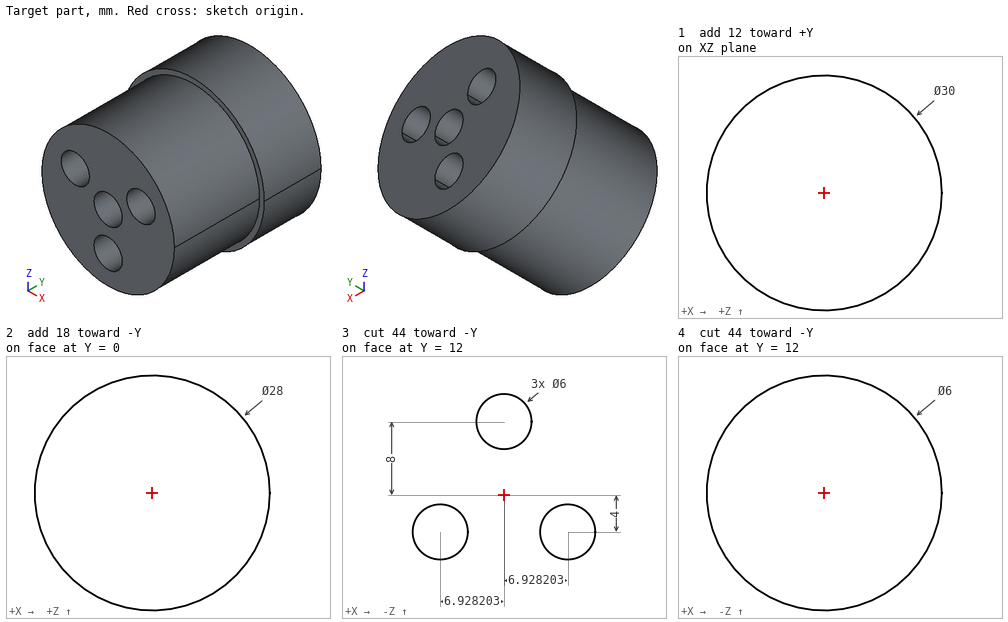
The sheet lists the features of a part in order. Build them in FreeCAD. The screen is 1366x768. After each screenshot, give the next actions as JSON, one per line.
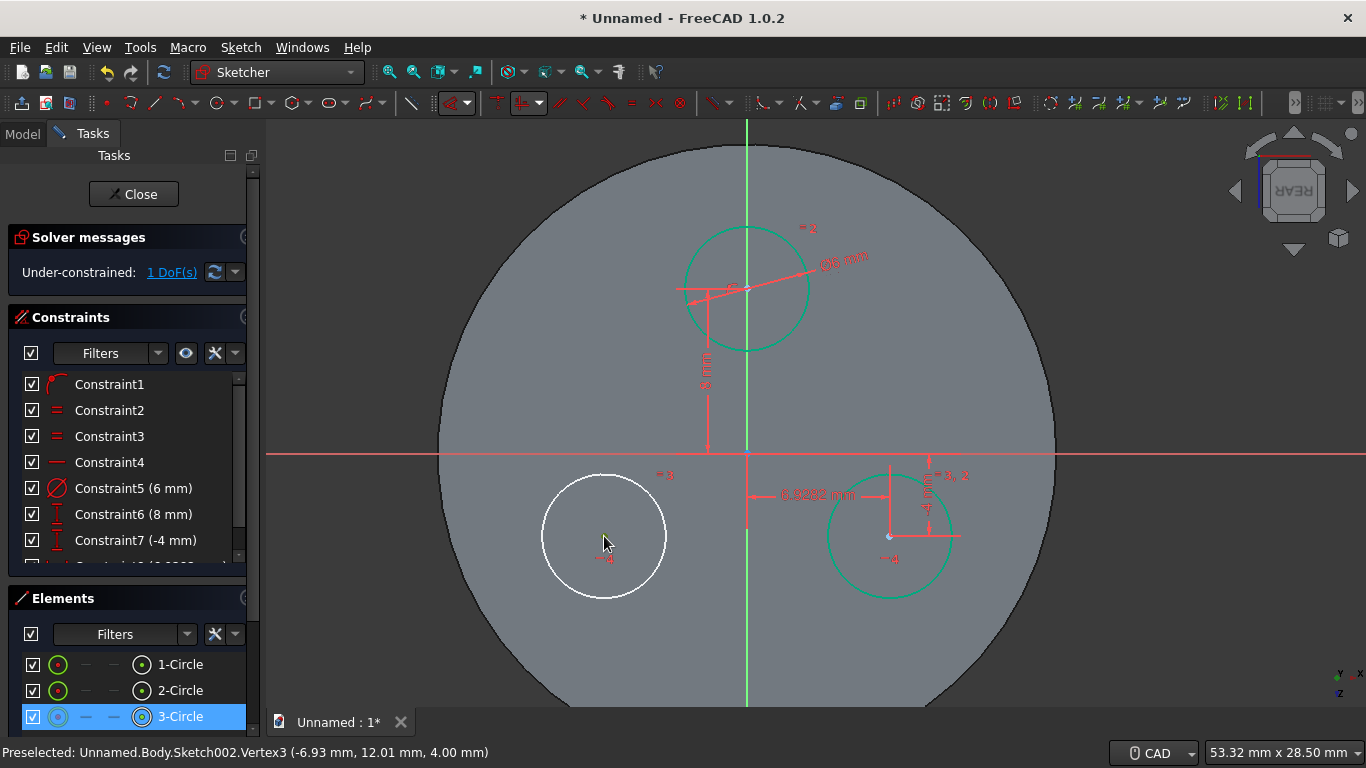
{"action": "left_click", "coordinate": [470, 104]}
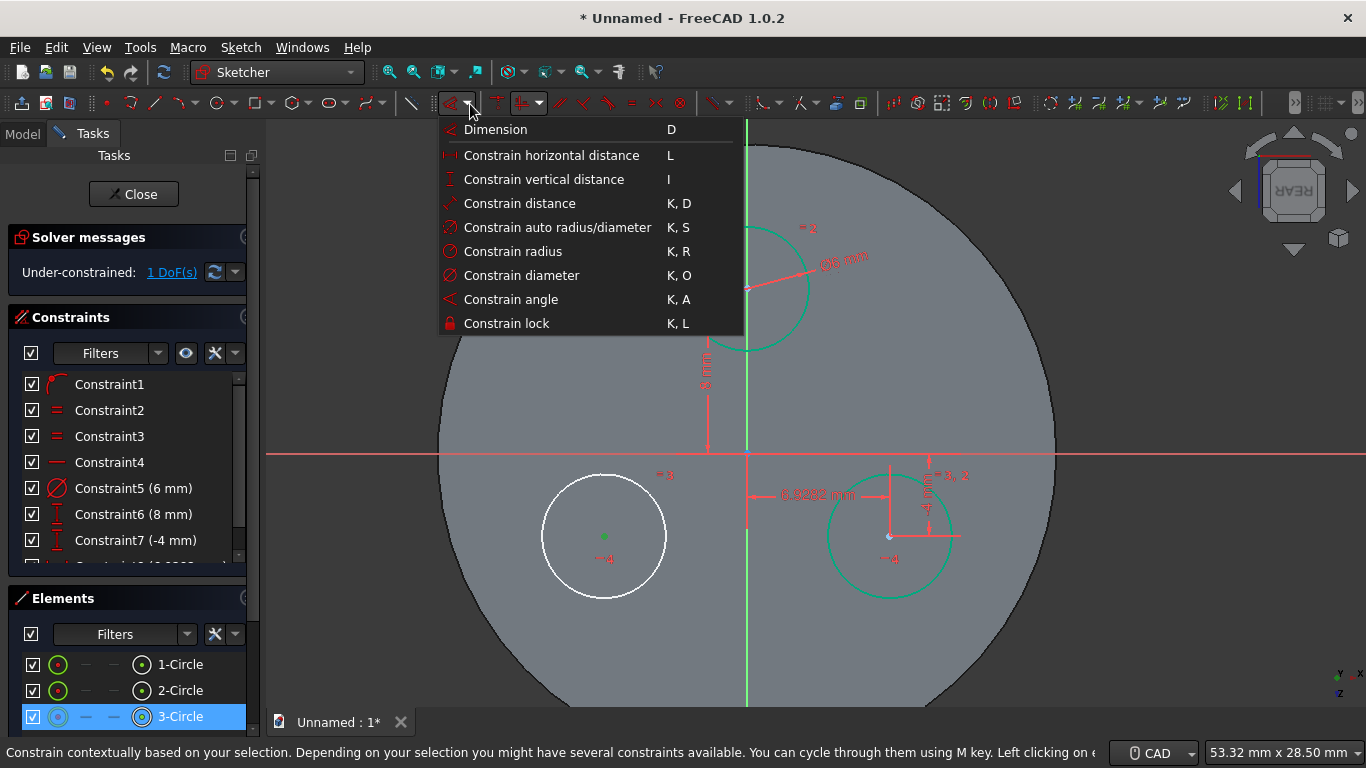
{"action": "left_click", "coordinate": [591, 155]}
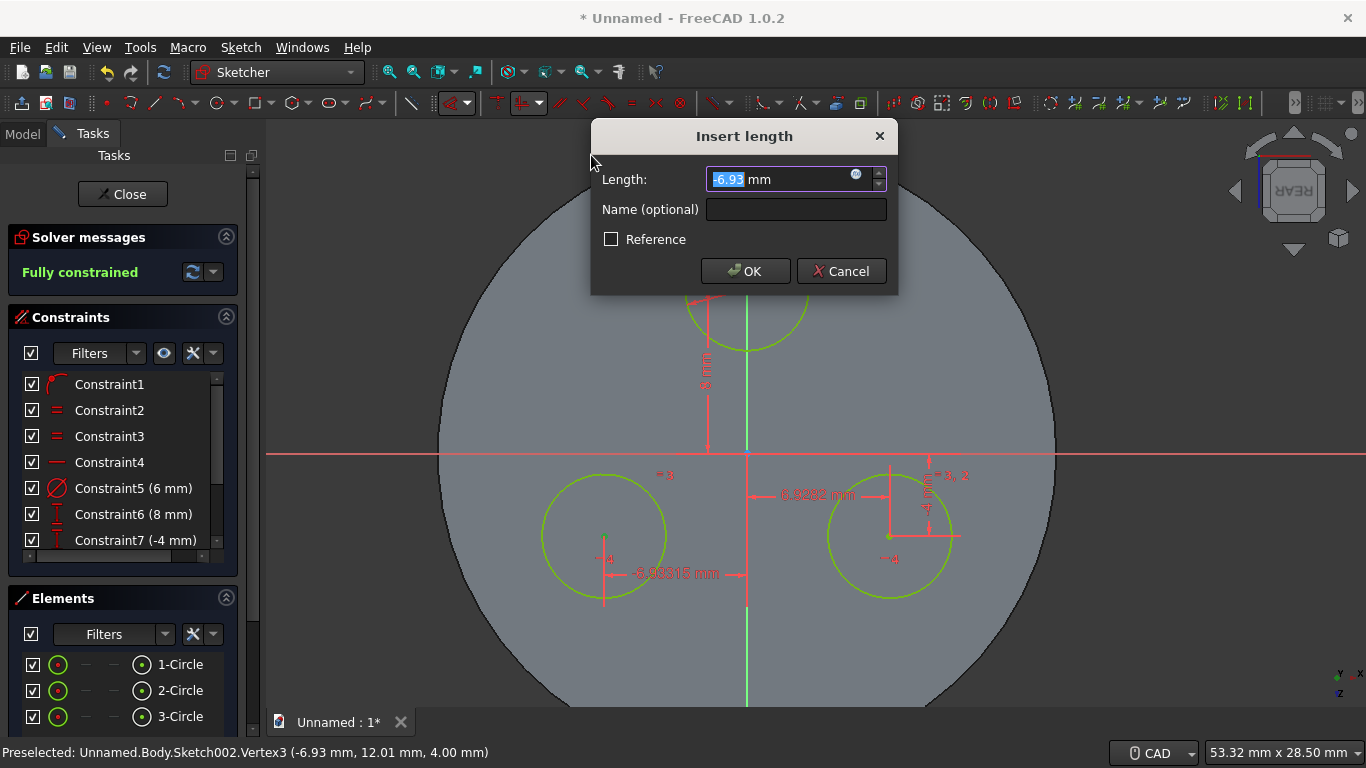
{"action": "type", "text": "-6.928203"}
{"action": "key", "text": "Return"}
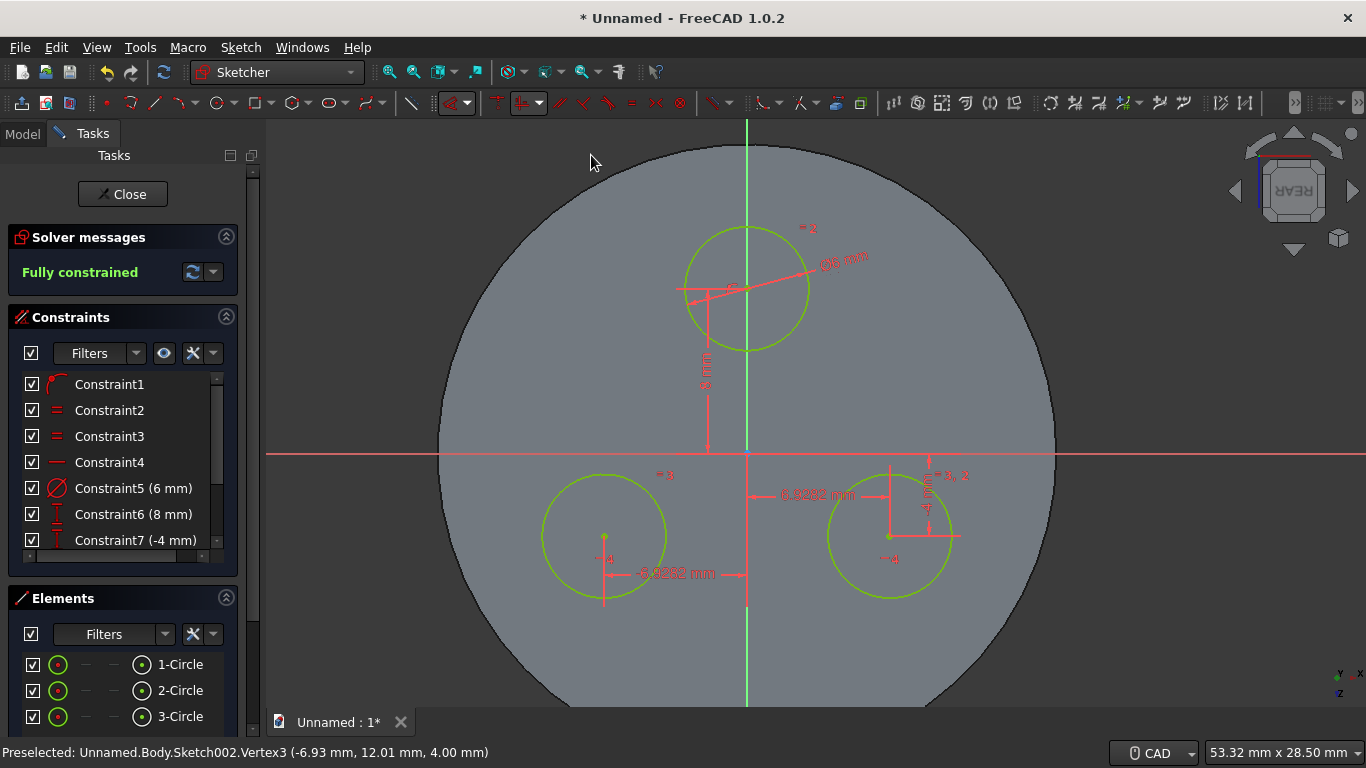
{"action": "left_click", "coordinate": [123, 194]}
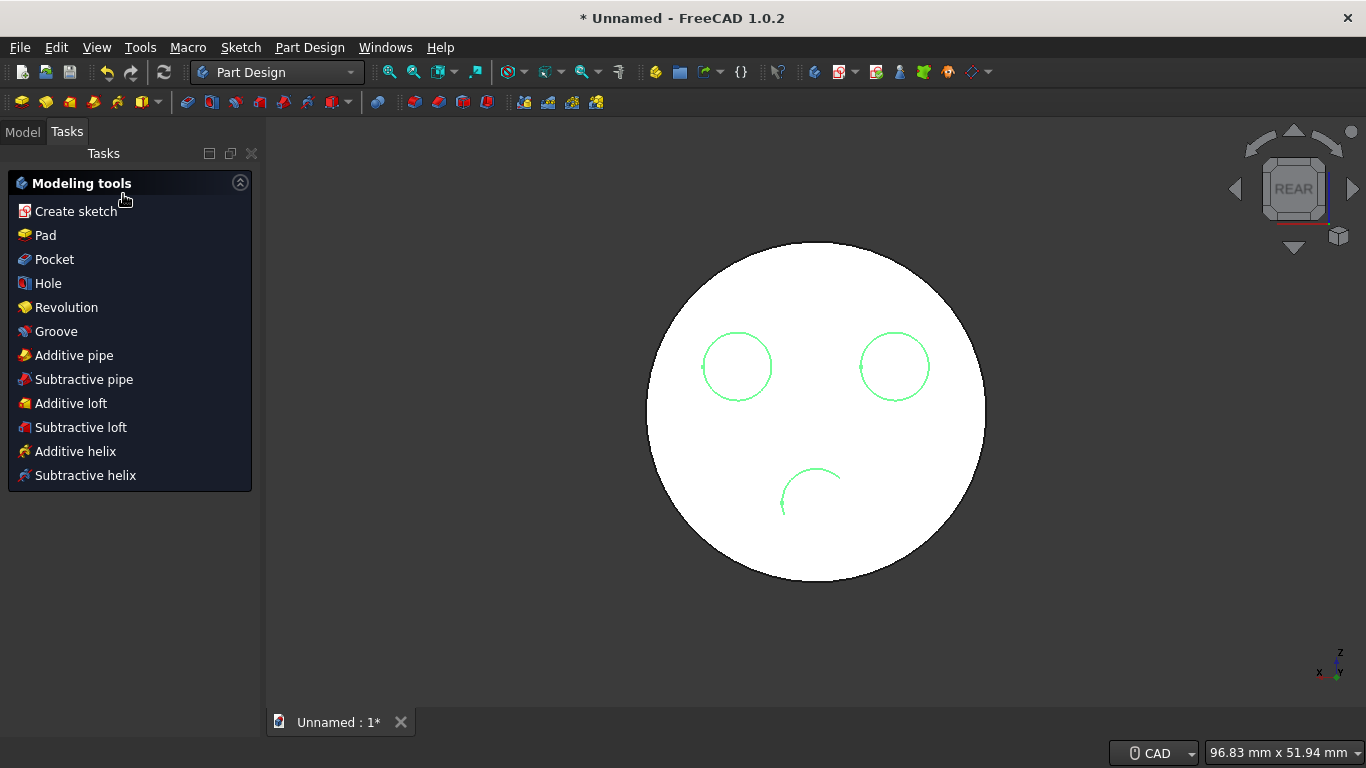
{"action": "left_click", "coordinate": [188, 102]}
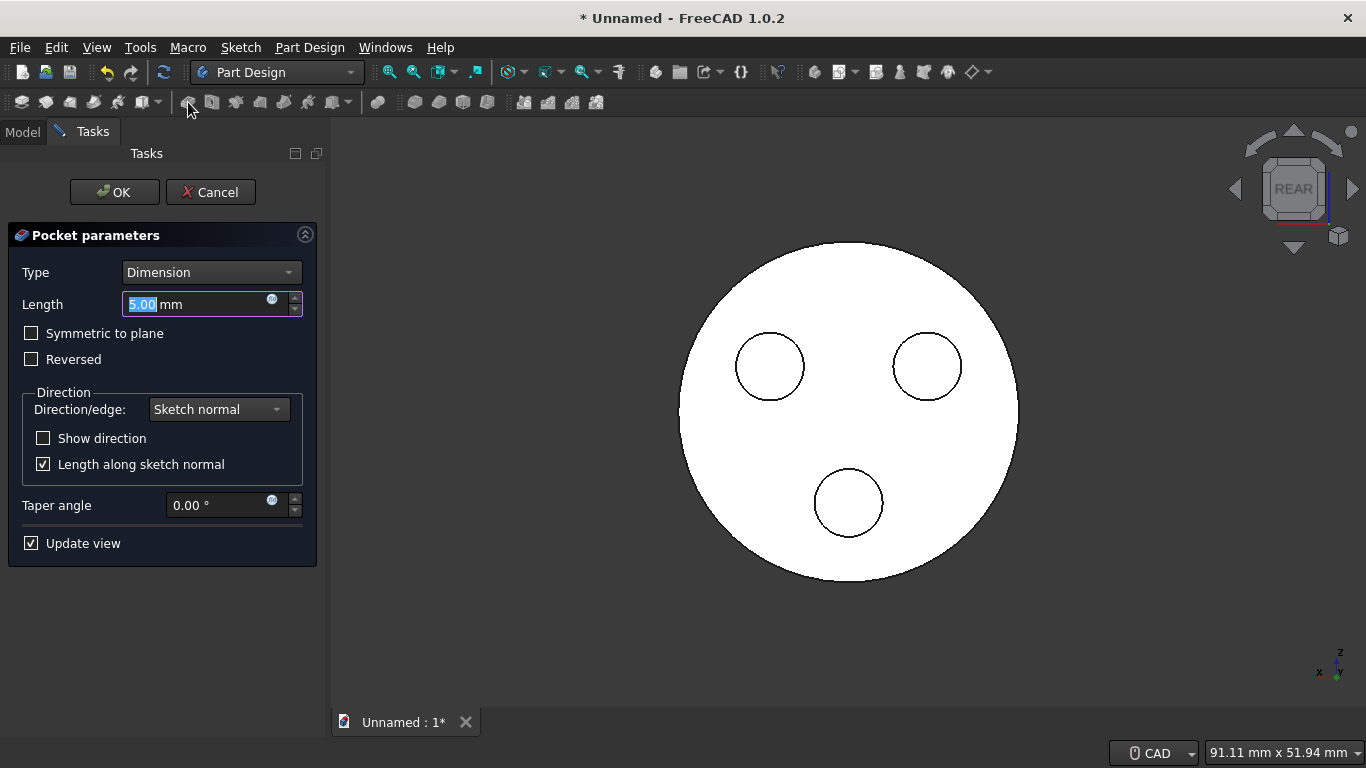
{"action": "type", "text": "44"}
{"action": "key", "text": "Tab"}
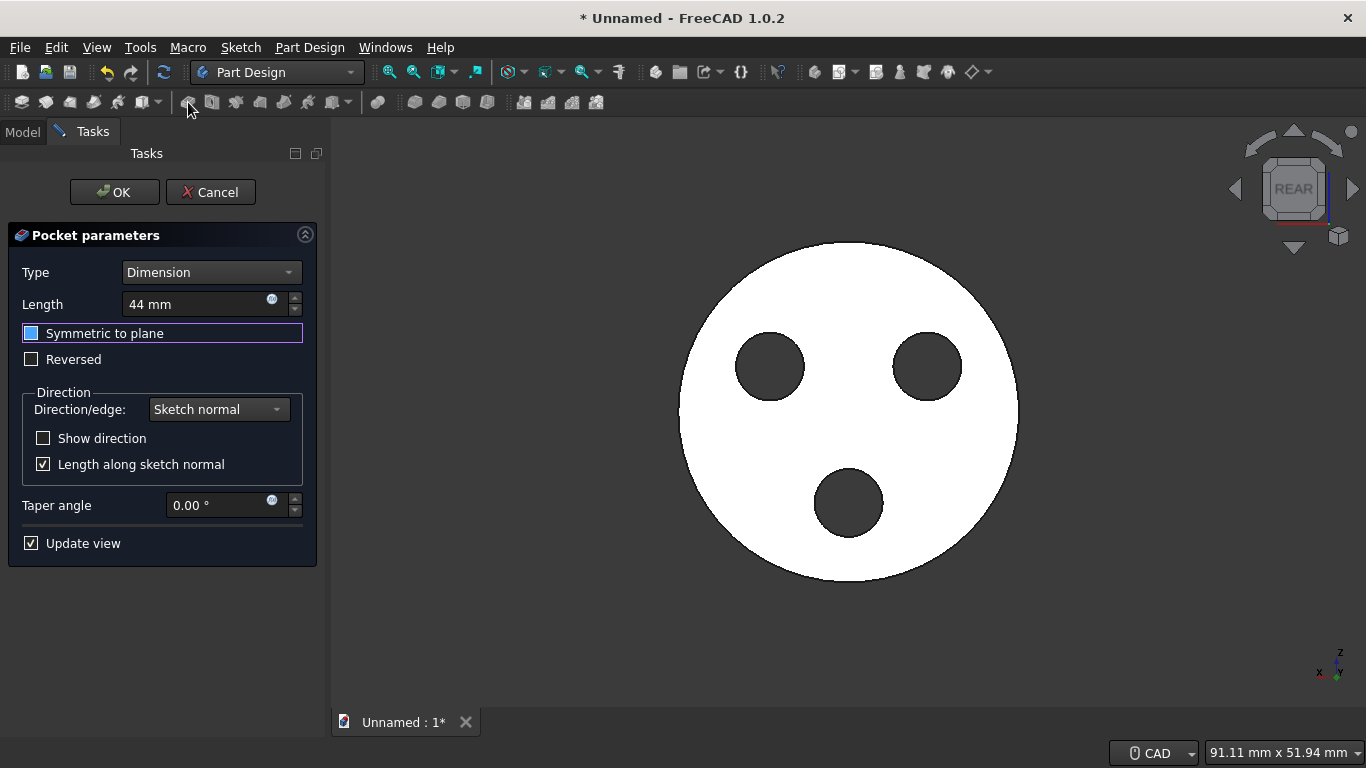
{"action": "left_click", "coordinate": [115, 192]}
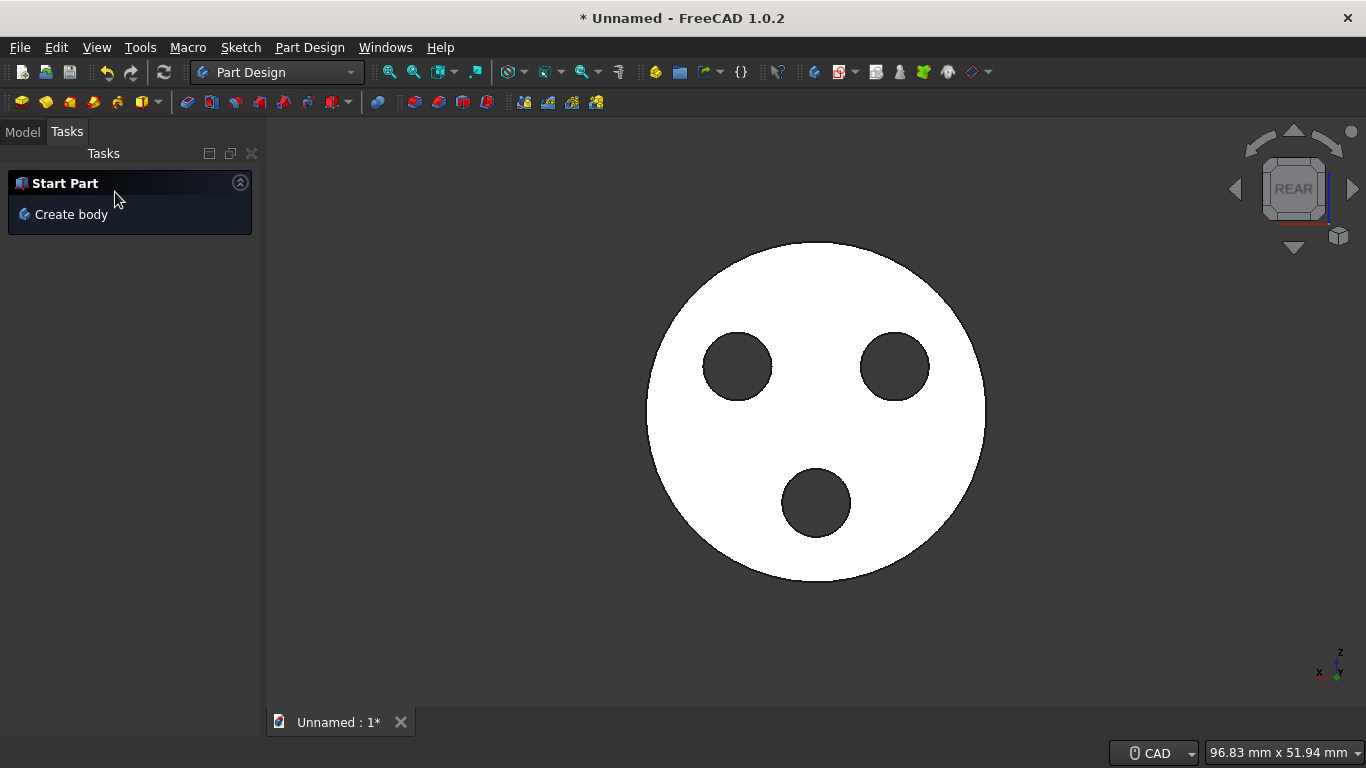
{"action": "left_click", "coordinate": [914, 460]}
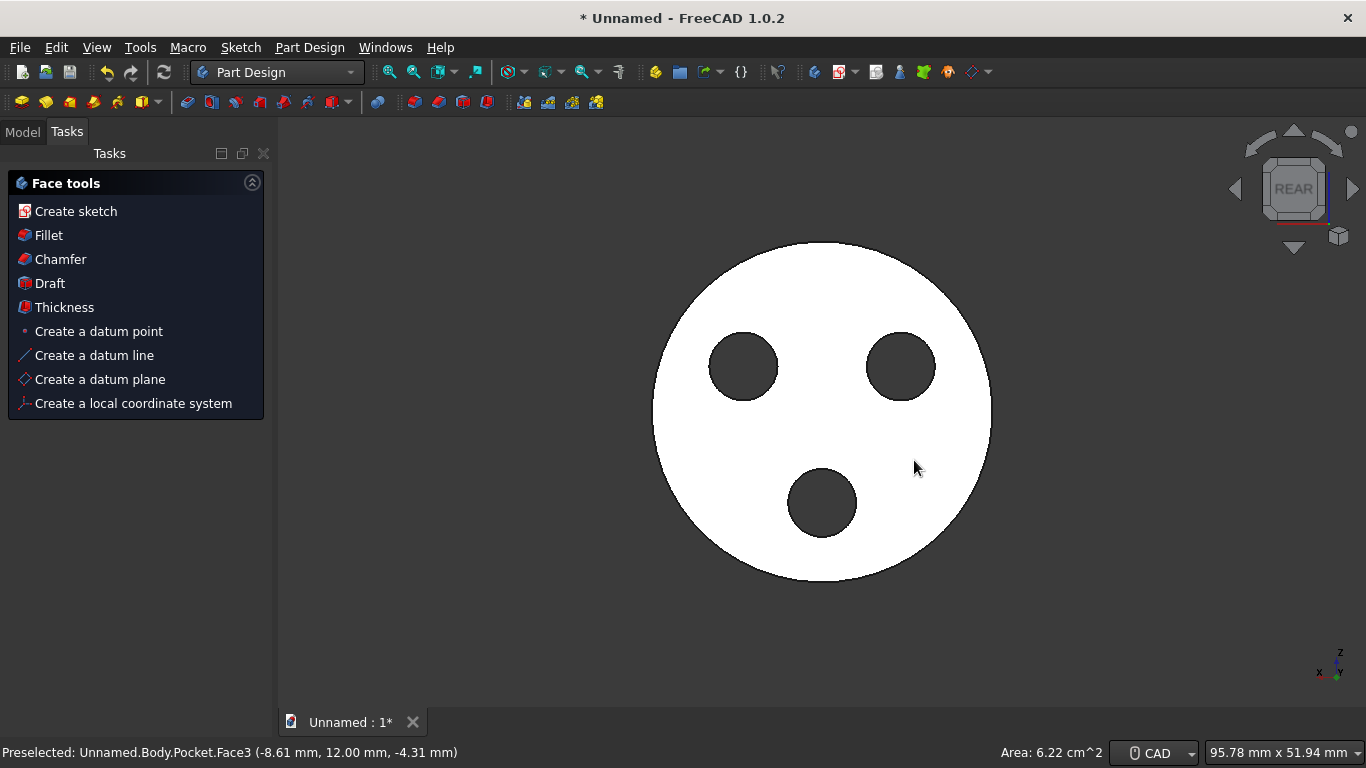
{"action": "left_click", "coordinate": [840, 72]}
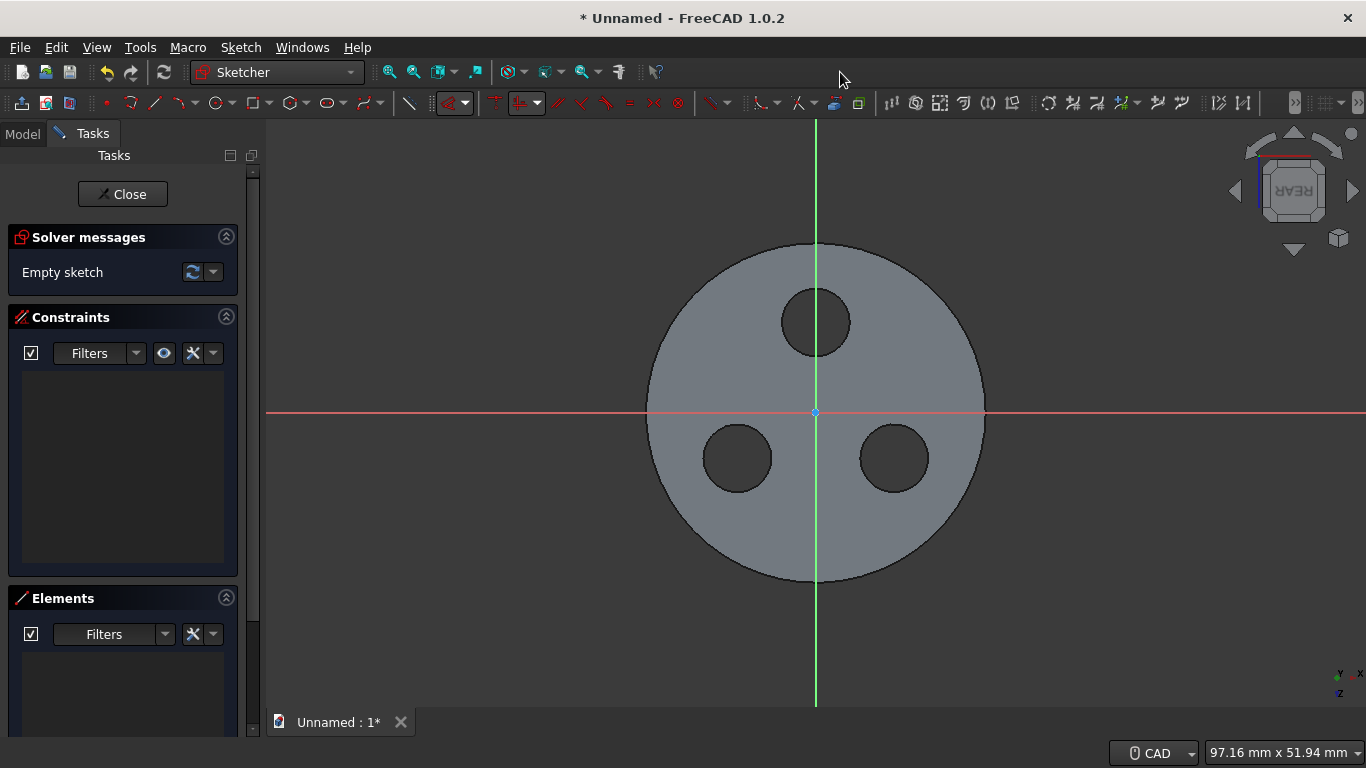
{"action": "scroll", "coordinate": [829, 413], "scroll_direction": "up", "scroll_amount": 9}